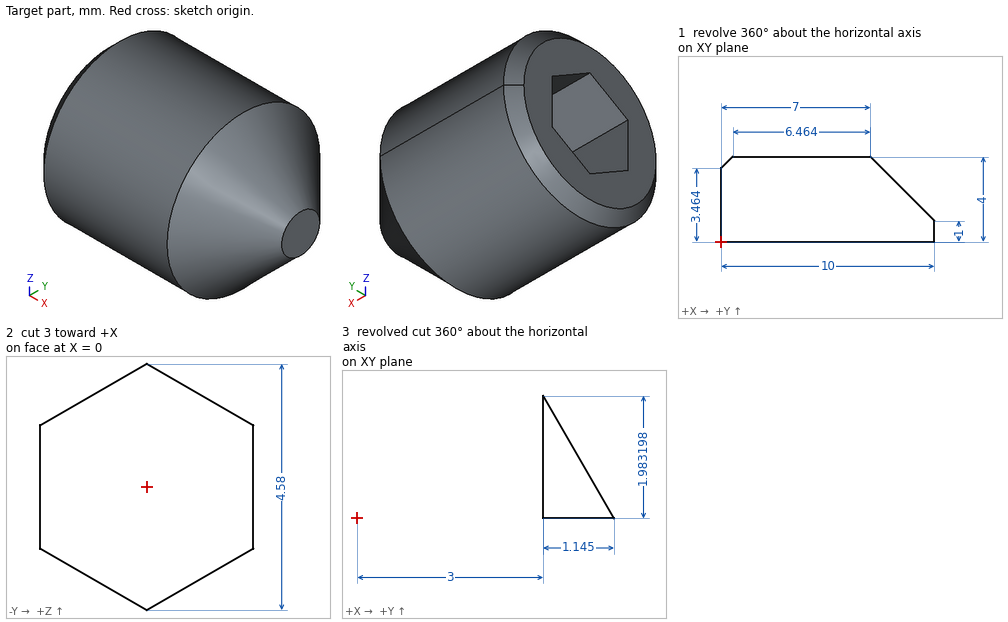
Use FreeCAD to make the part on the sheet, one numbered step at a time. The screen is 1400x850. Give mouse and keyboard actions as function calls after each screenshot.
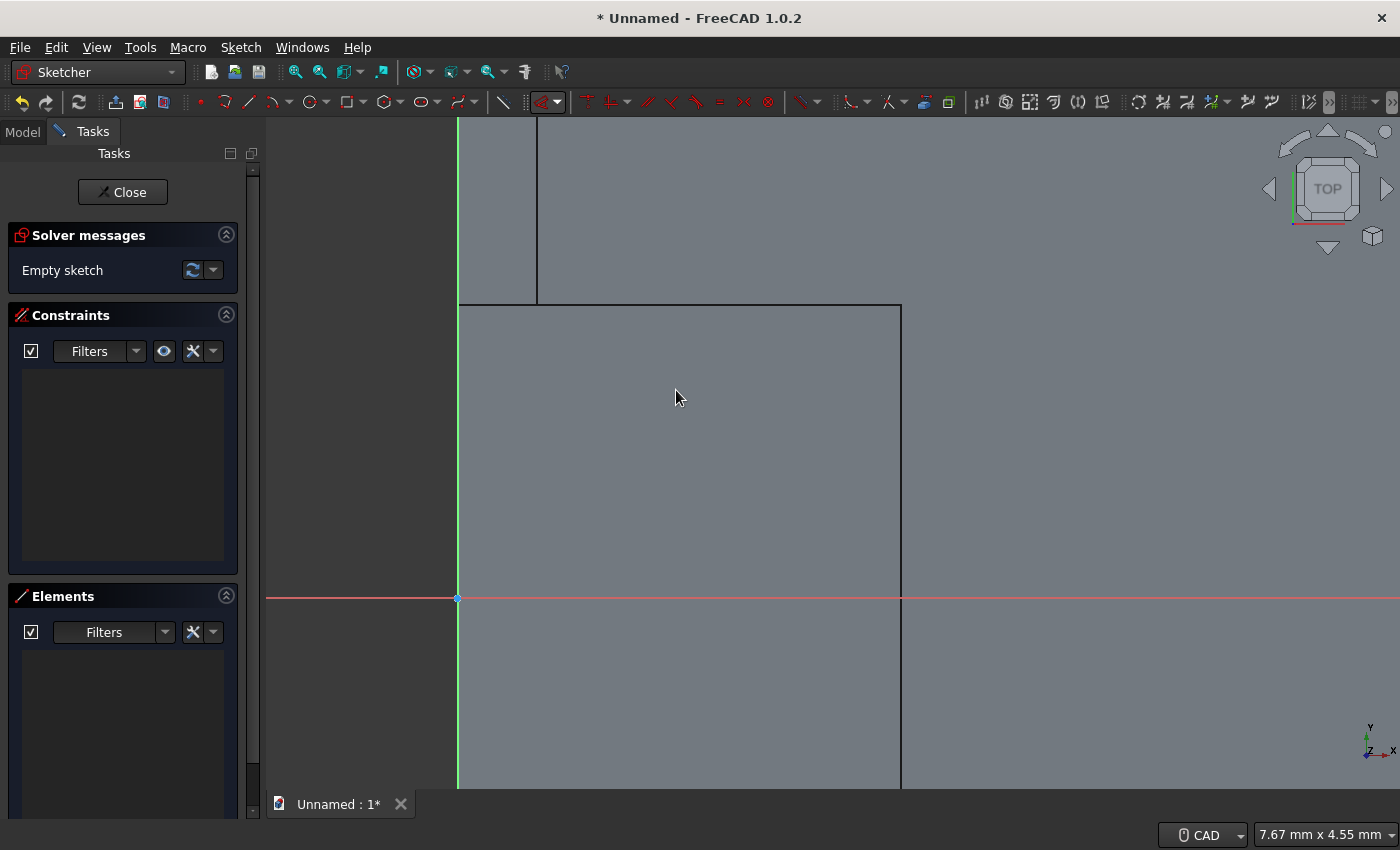
click(226, 102)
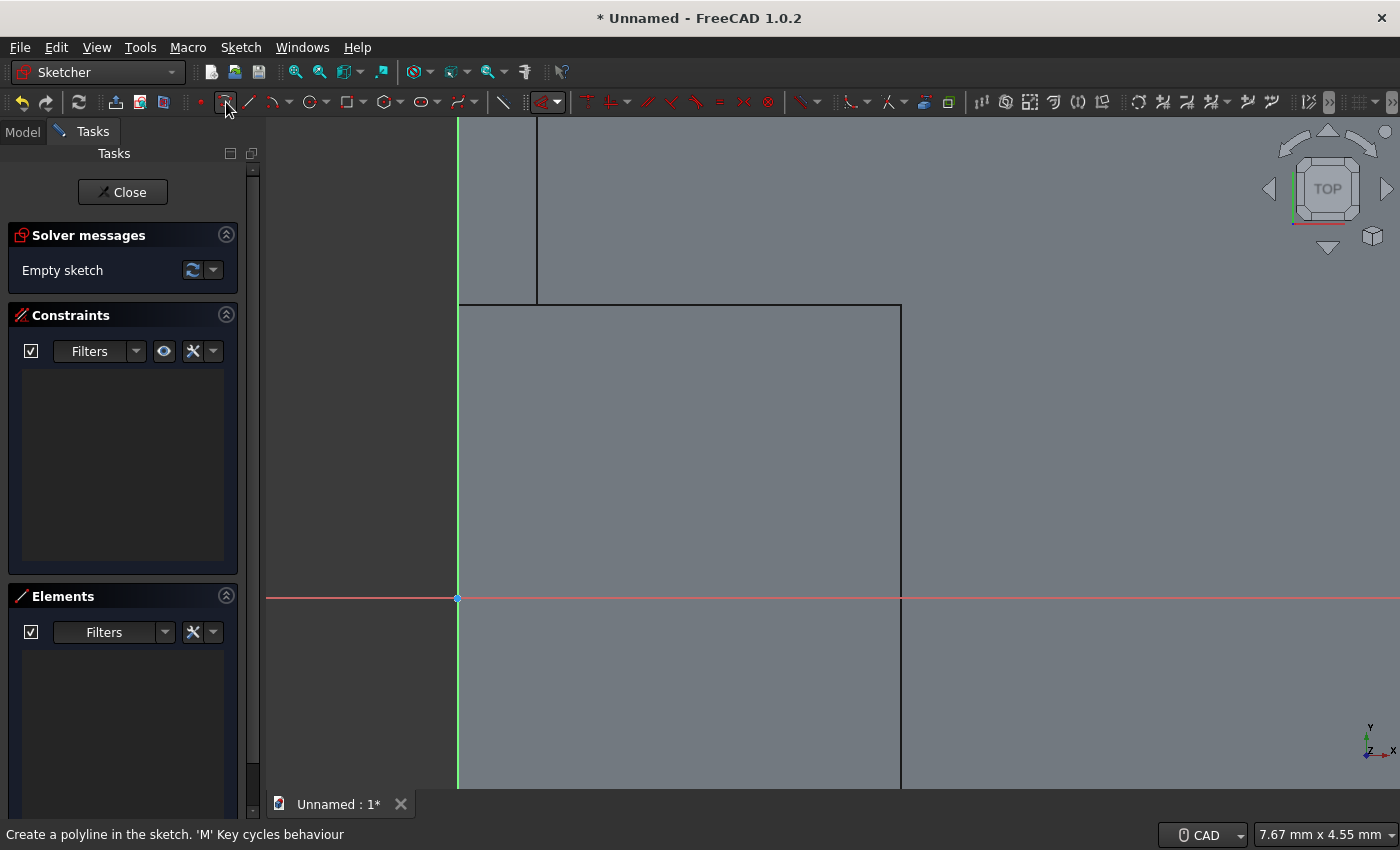
click(901, 598)
click(1070, 589)
click(901, 305)
click(901, 598)
key(Escape)
key(Escape)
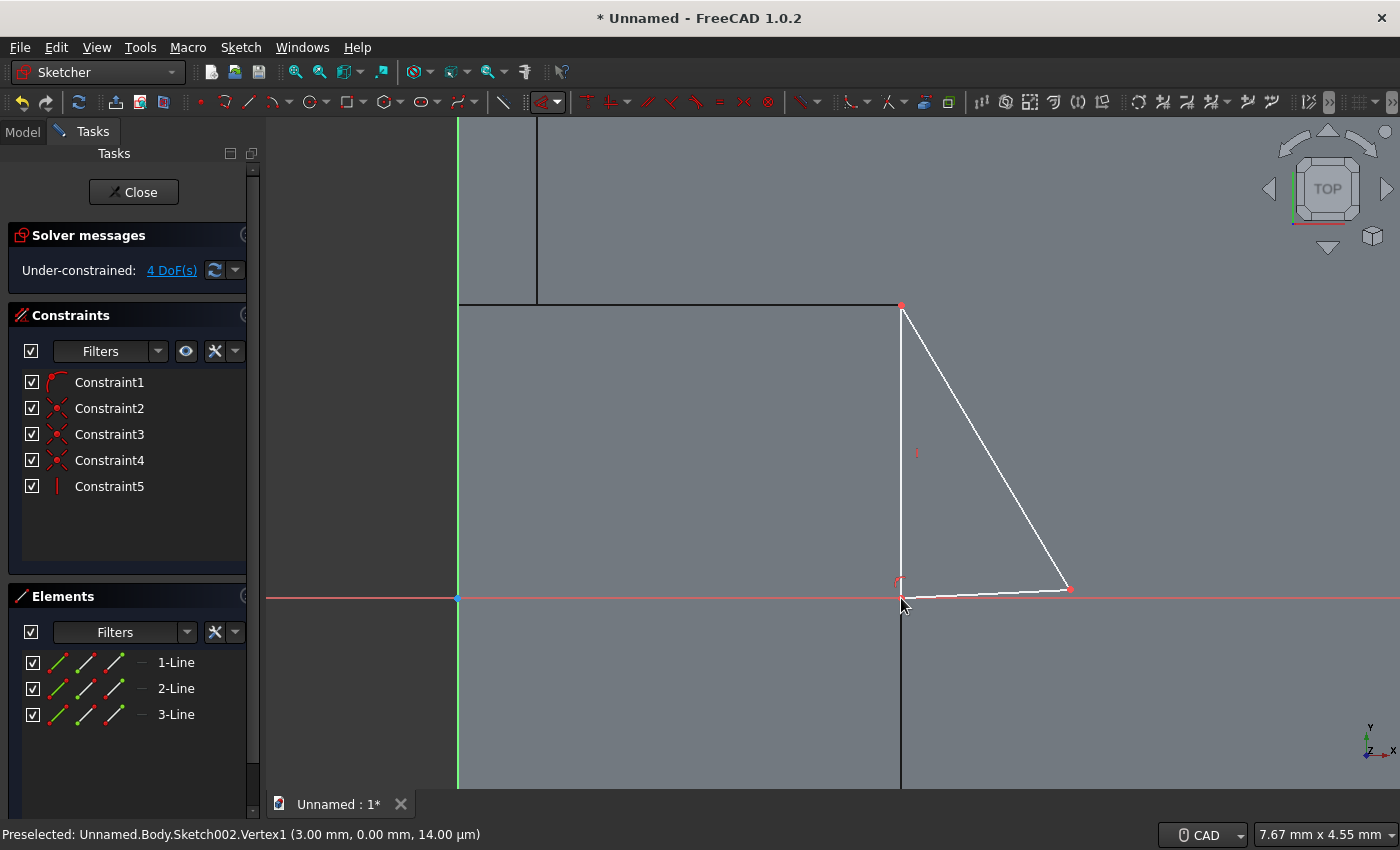
click(952, 596)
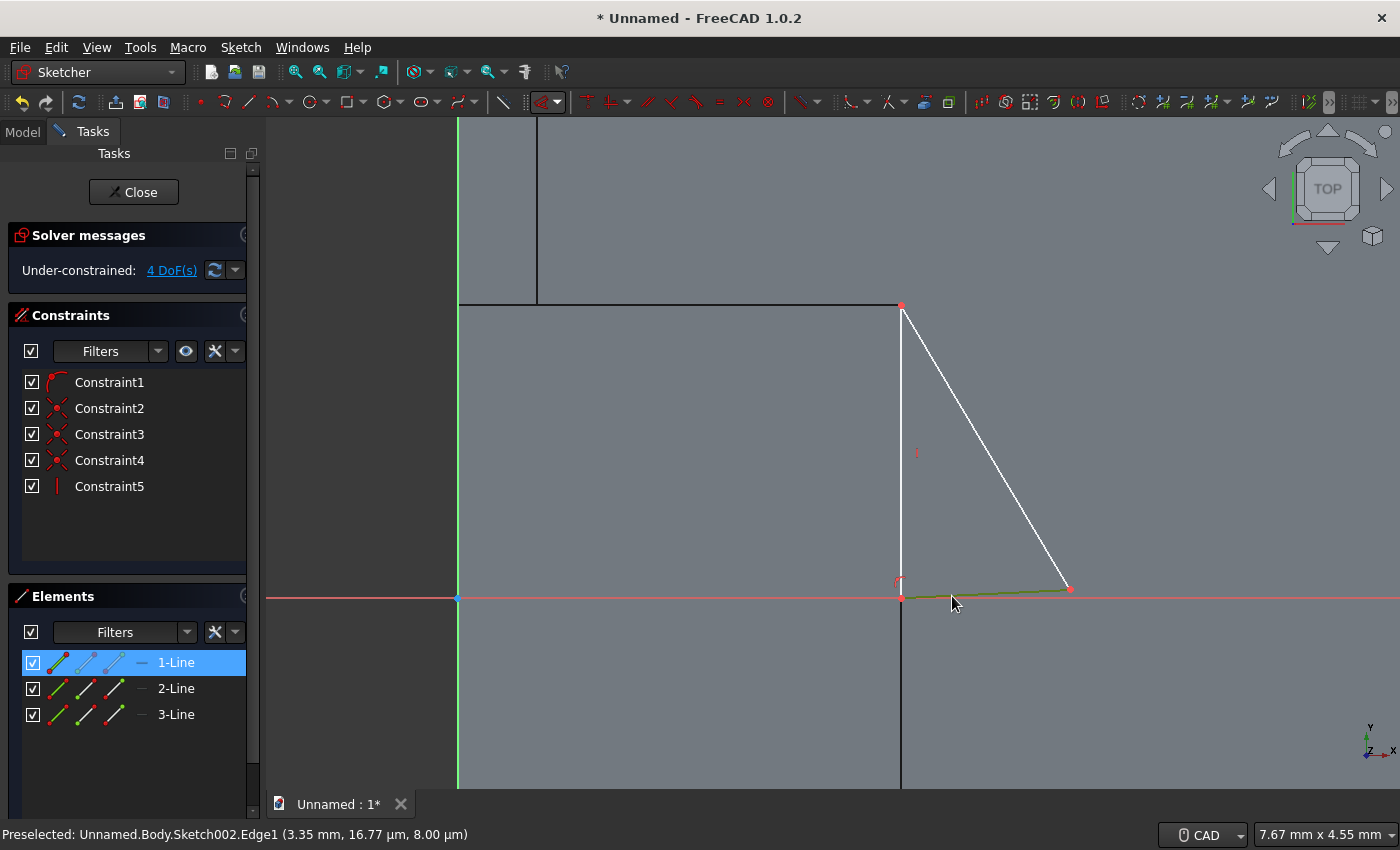
click(630, 102)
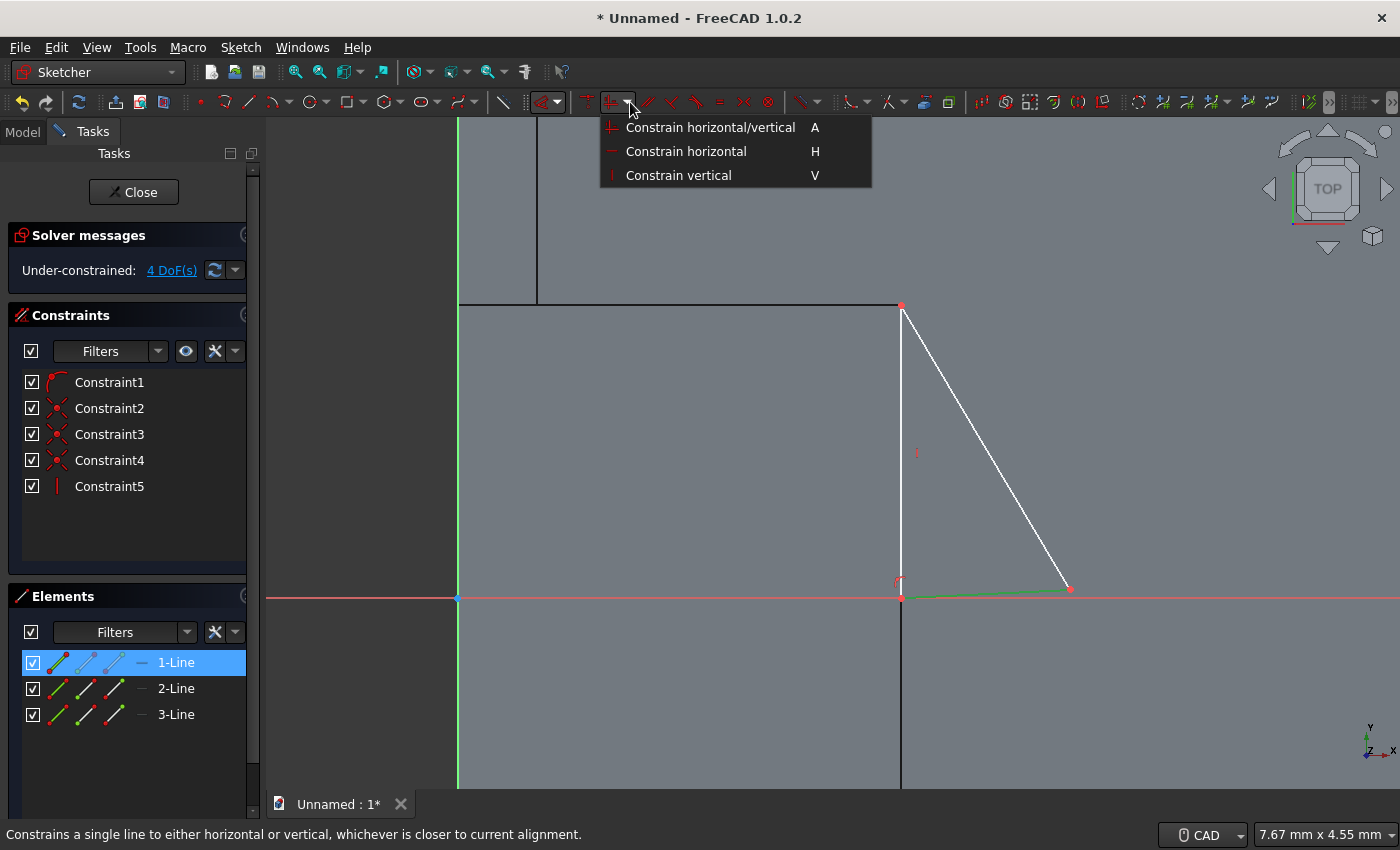
click(736, 151)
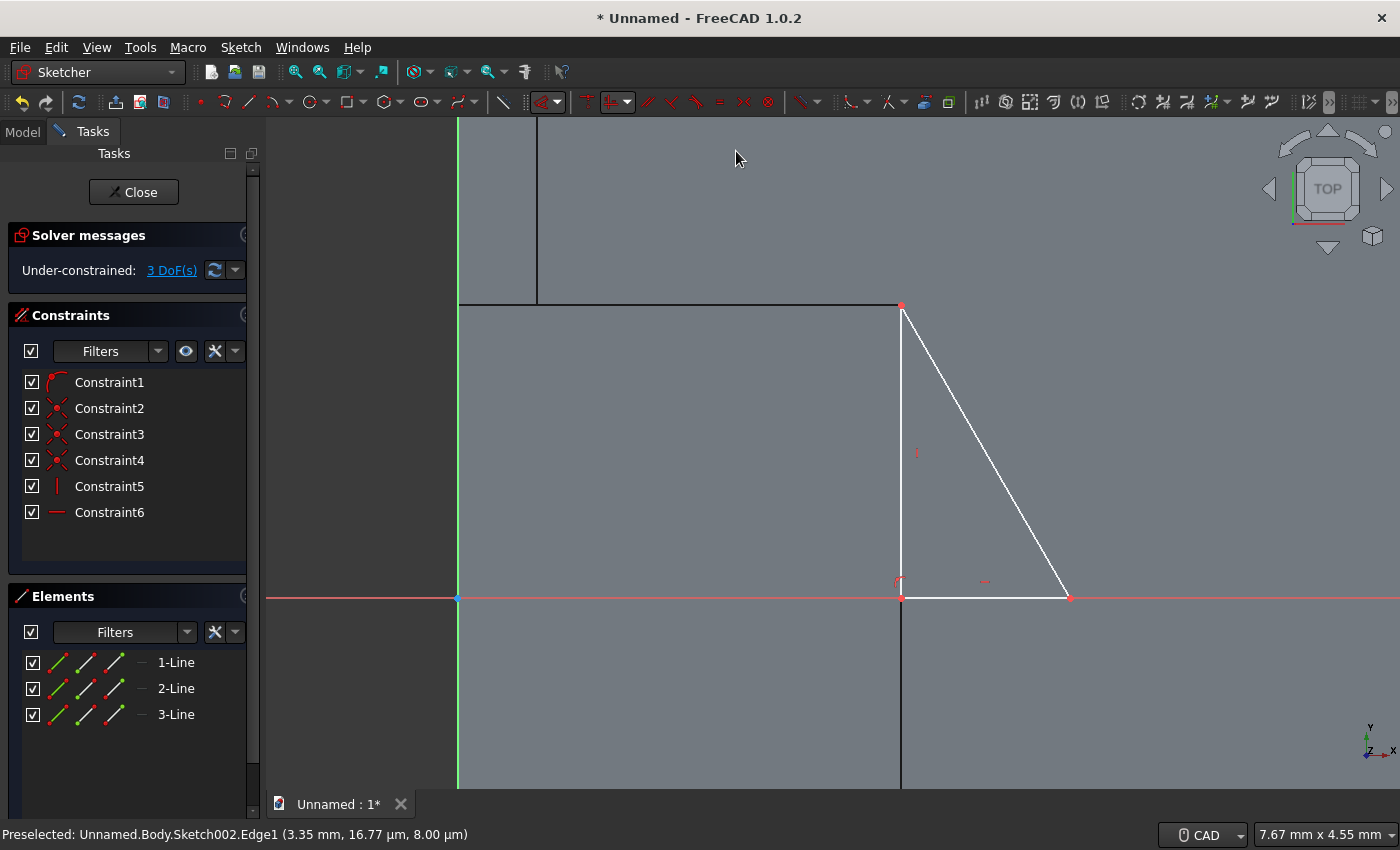
click(901, 598)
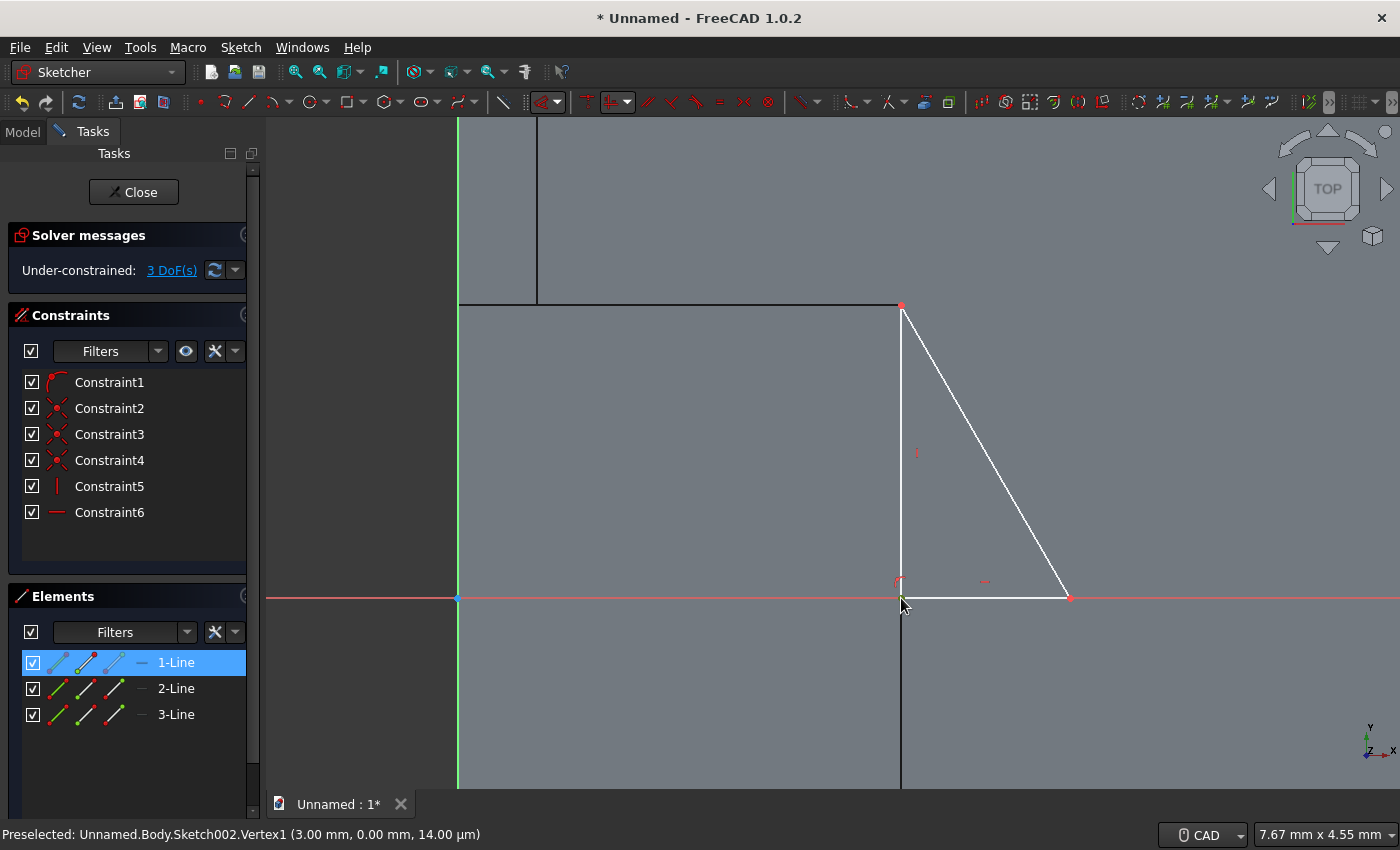
click(560, 102)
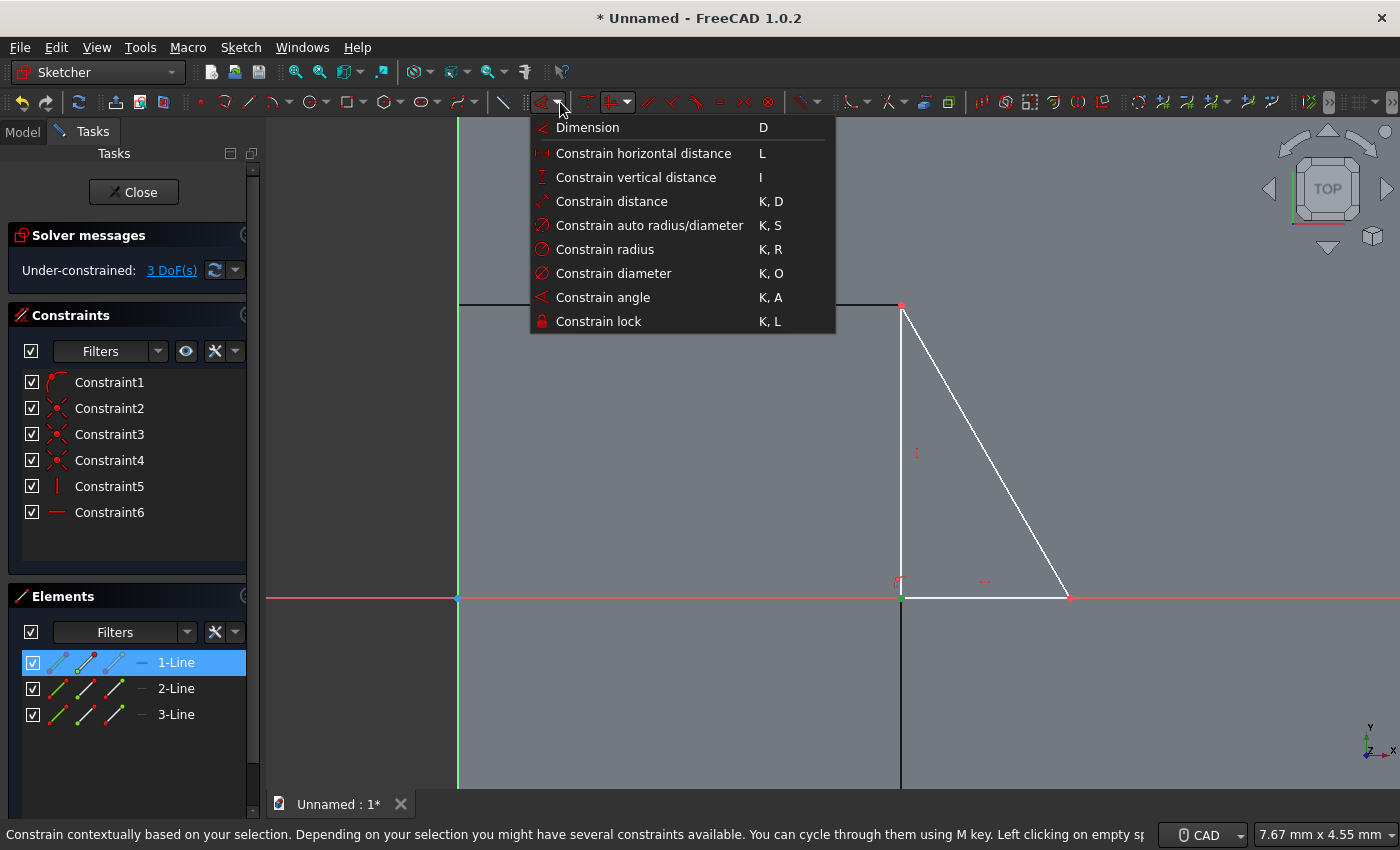
click(683, 153)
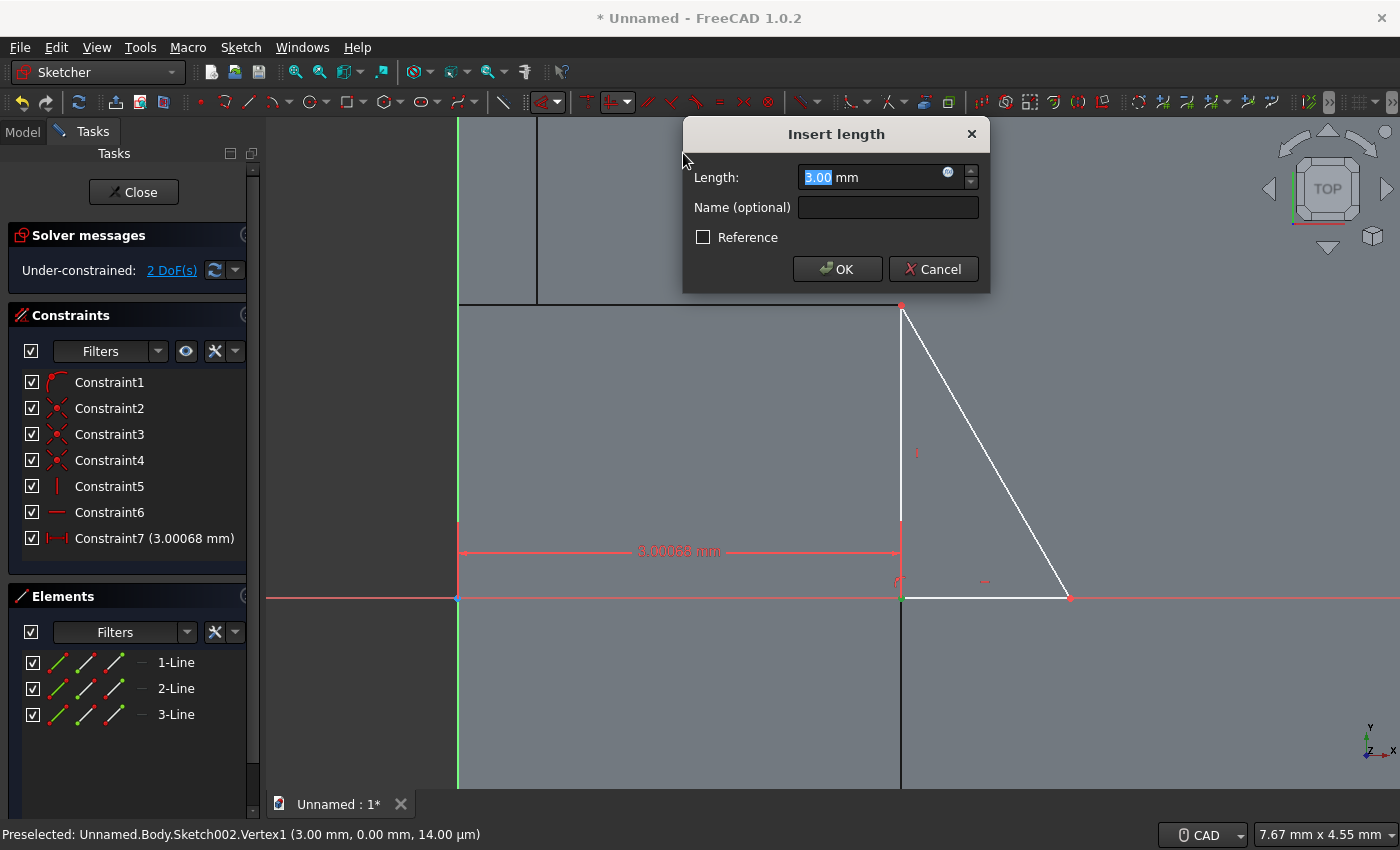
text(3)
key(Return)